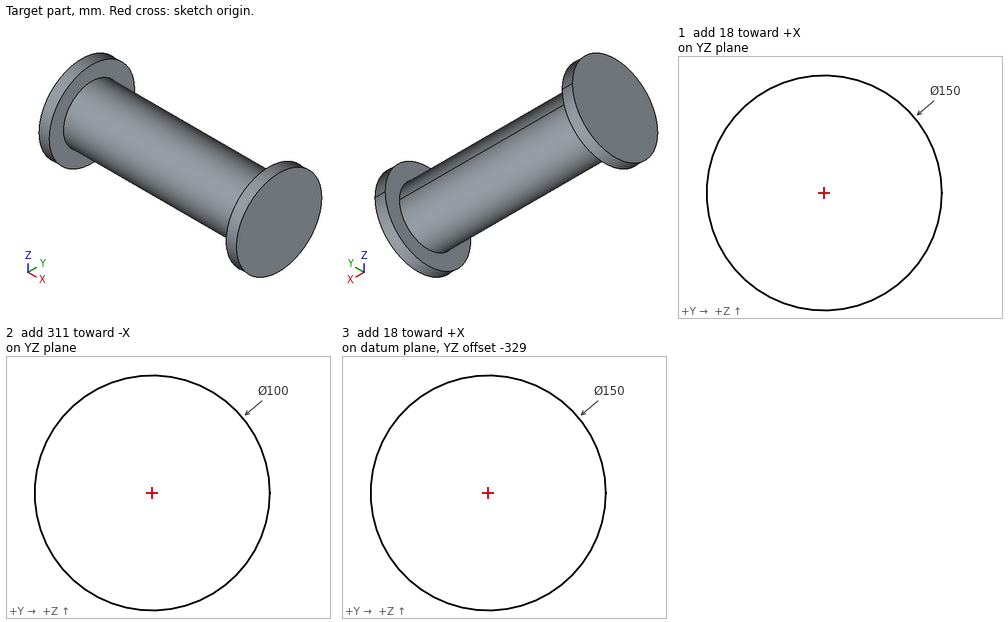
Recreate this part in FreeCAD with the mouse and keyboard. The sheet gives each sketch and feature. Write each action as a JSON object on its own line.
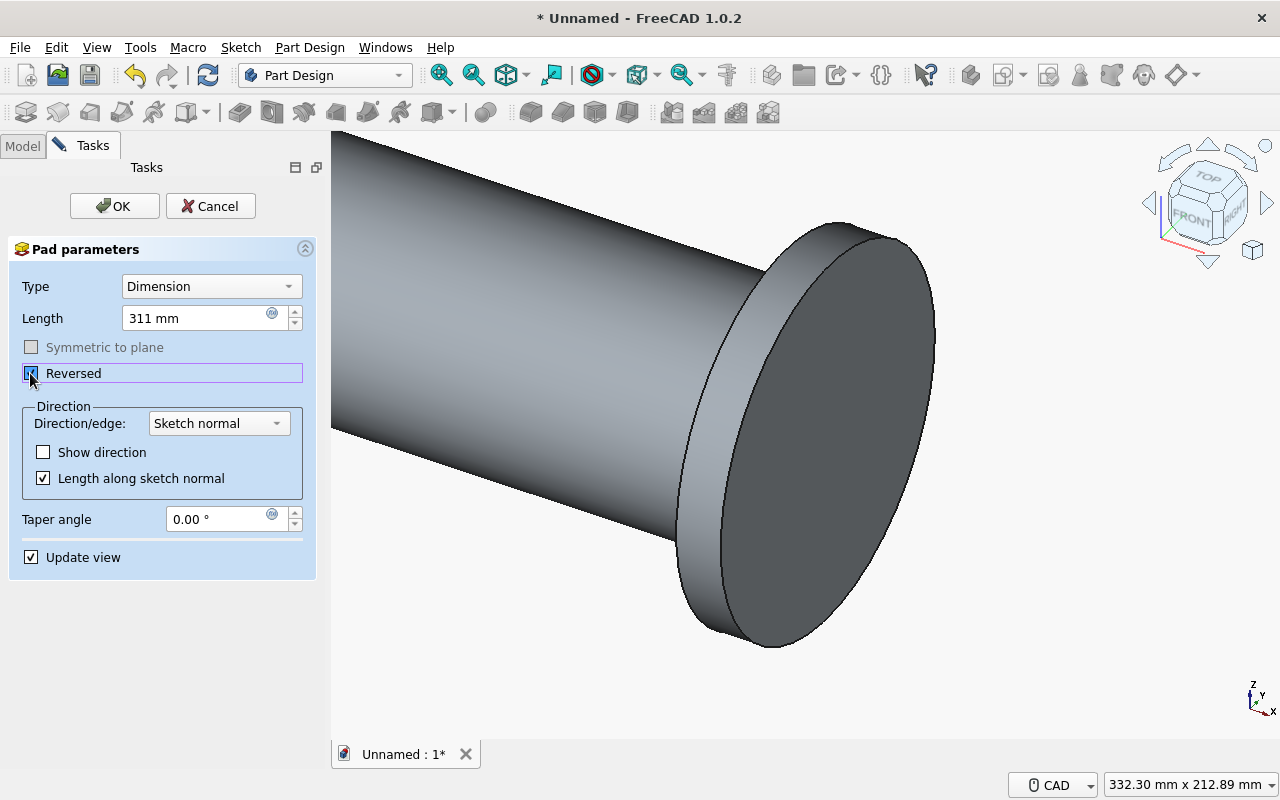
{"action": "left_click", "coordinate": [115, 206]}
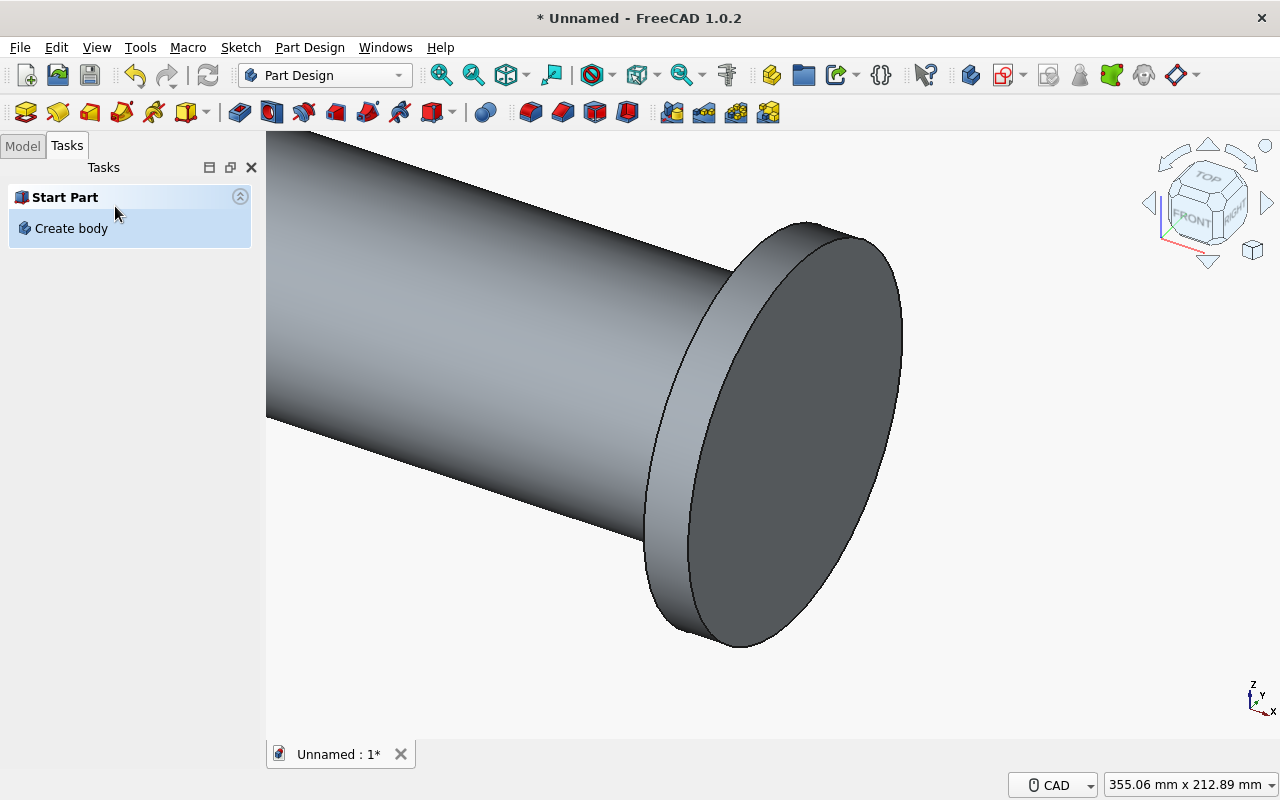
{"action": "left_click", "coordinate": [442, 76]}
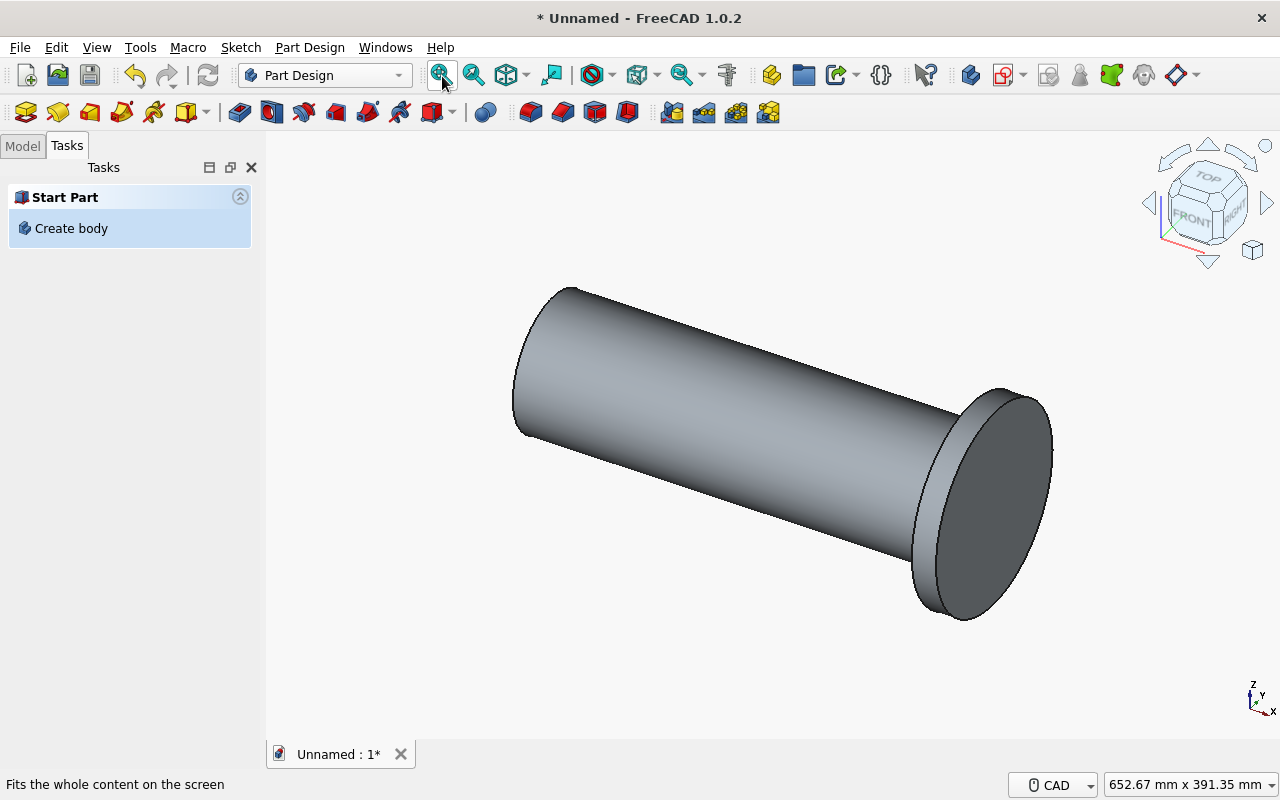
{"action": "left_click", "coordinate": [23, 145]}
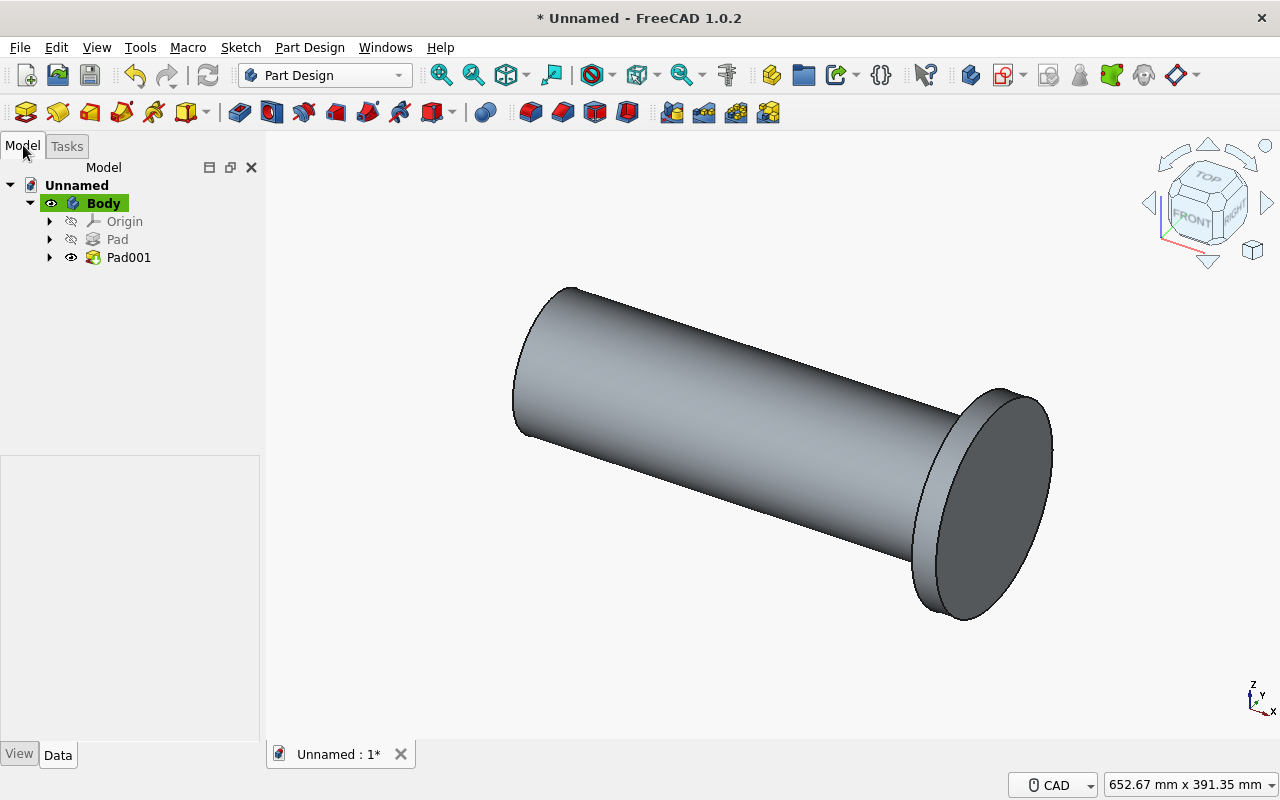
{"action": "left_click", "coordinate": [50, 221]}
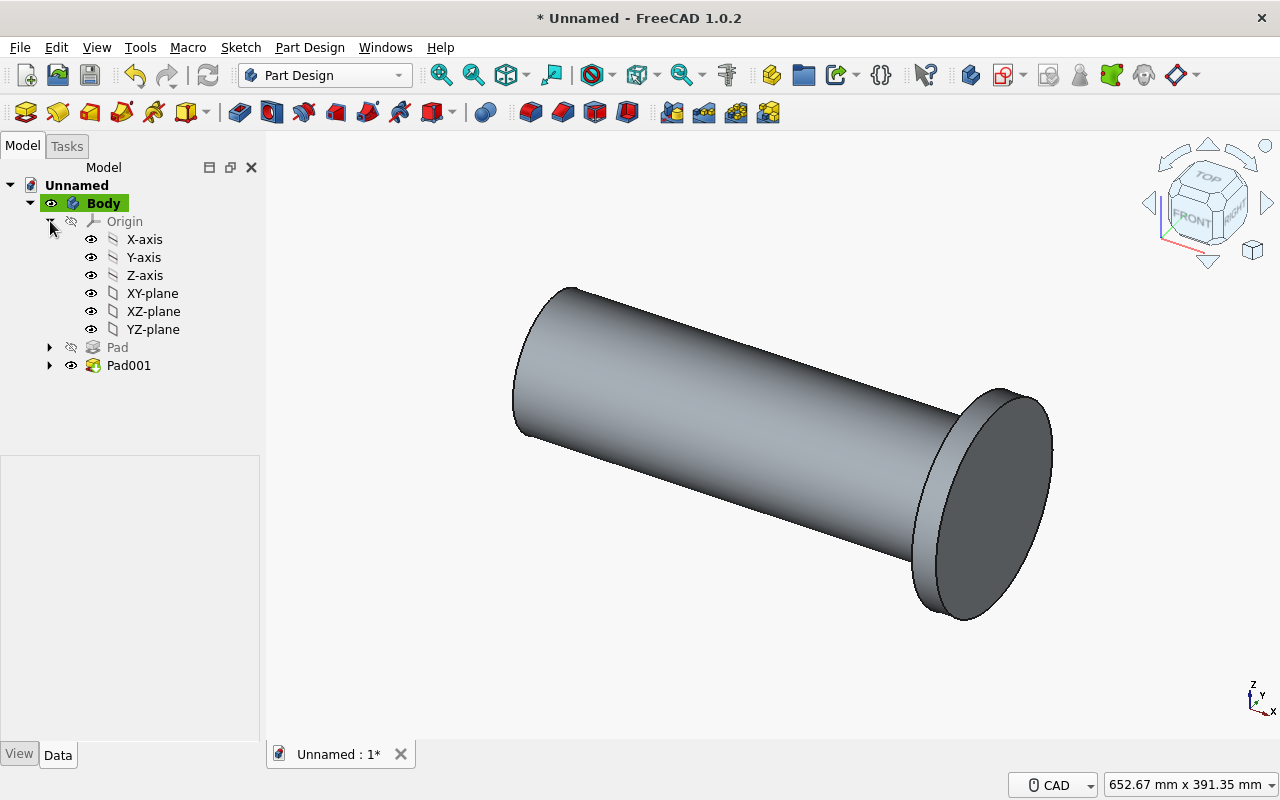
{"action": "left_click", "coordinate": [136, 329]}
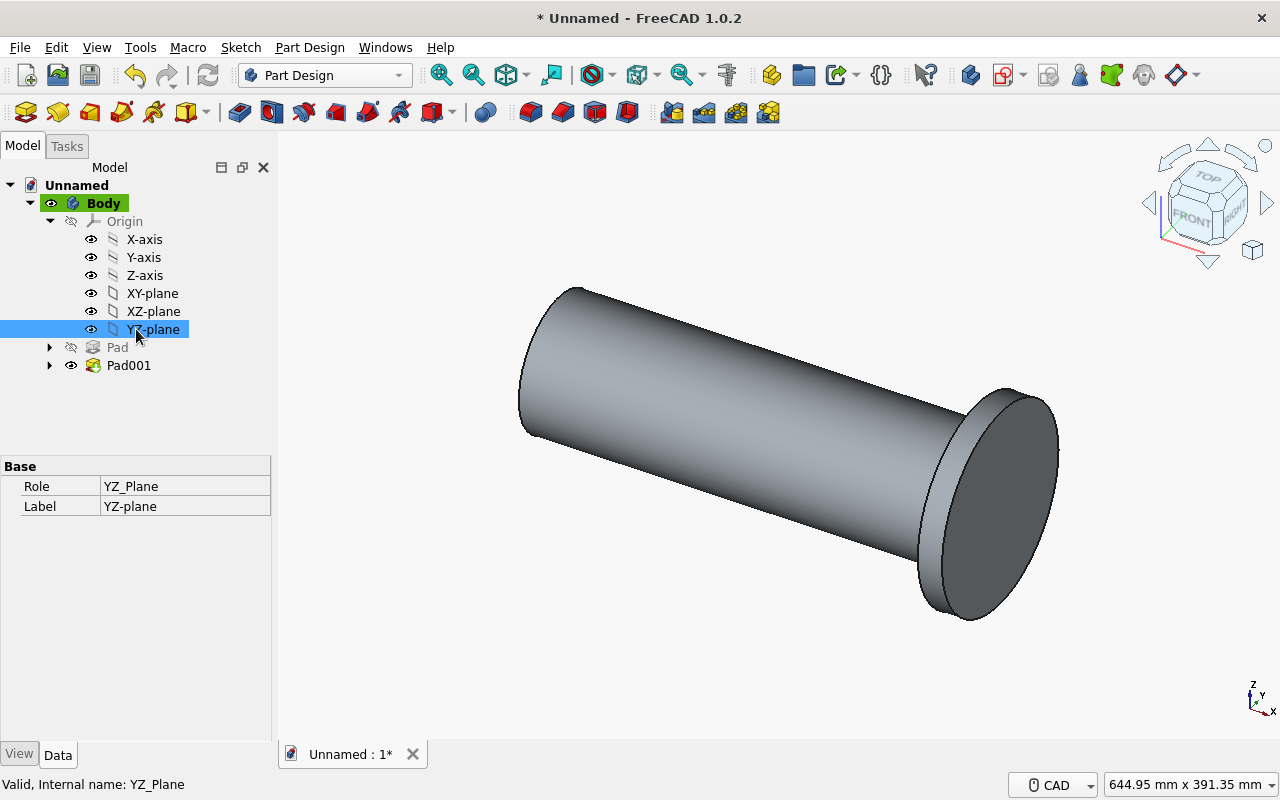
{"action": "left_click", "coordinate": [1176, 76]}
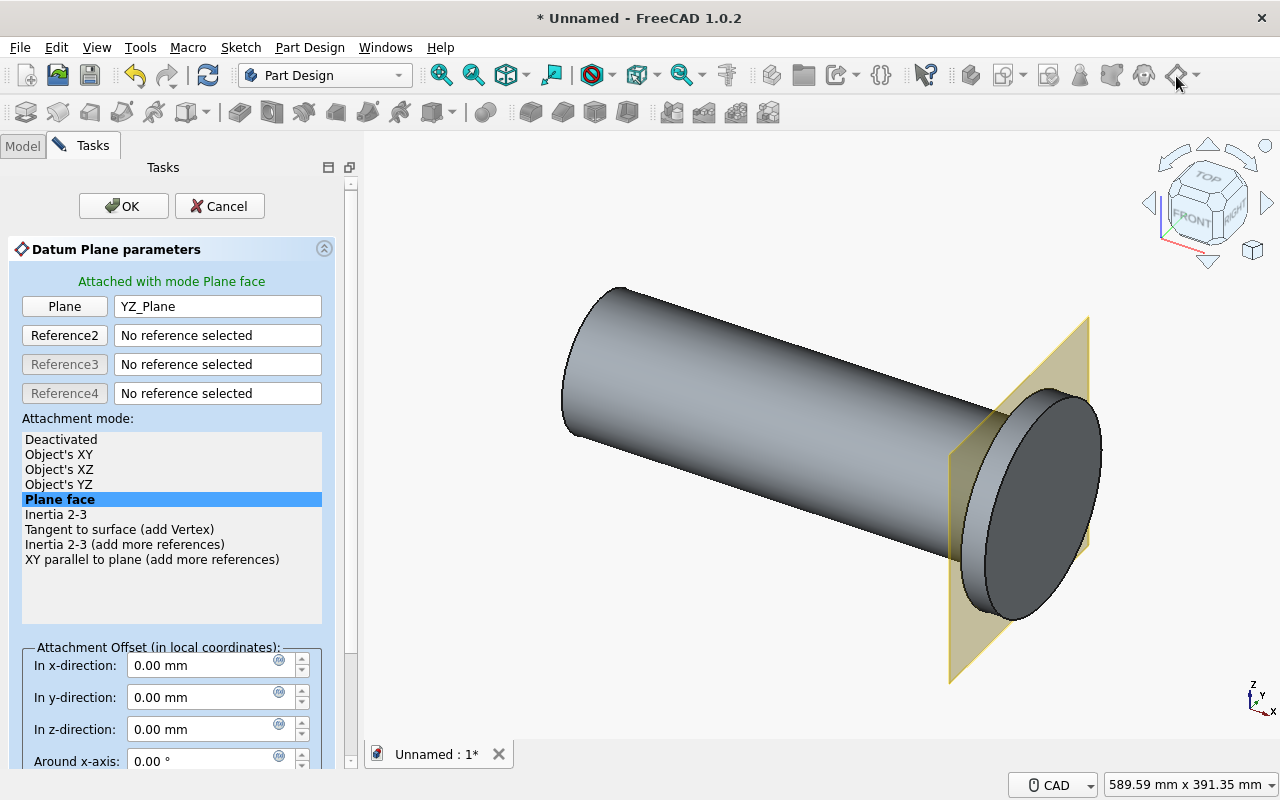
{"action": "triple_click", "coordinate": [210, 729]}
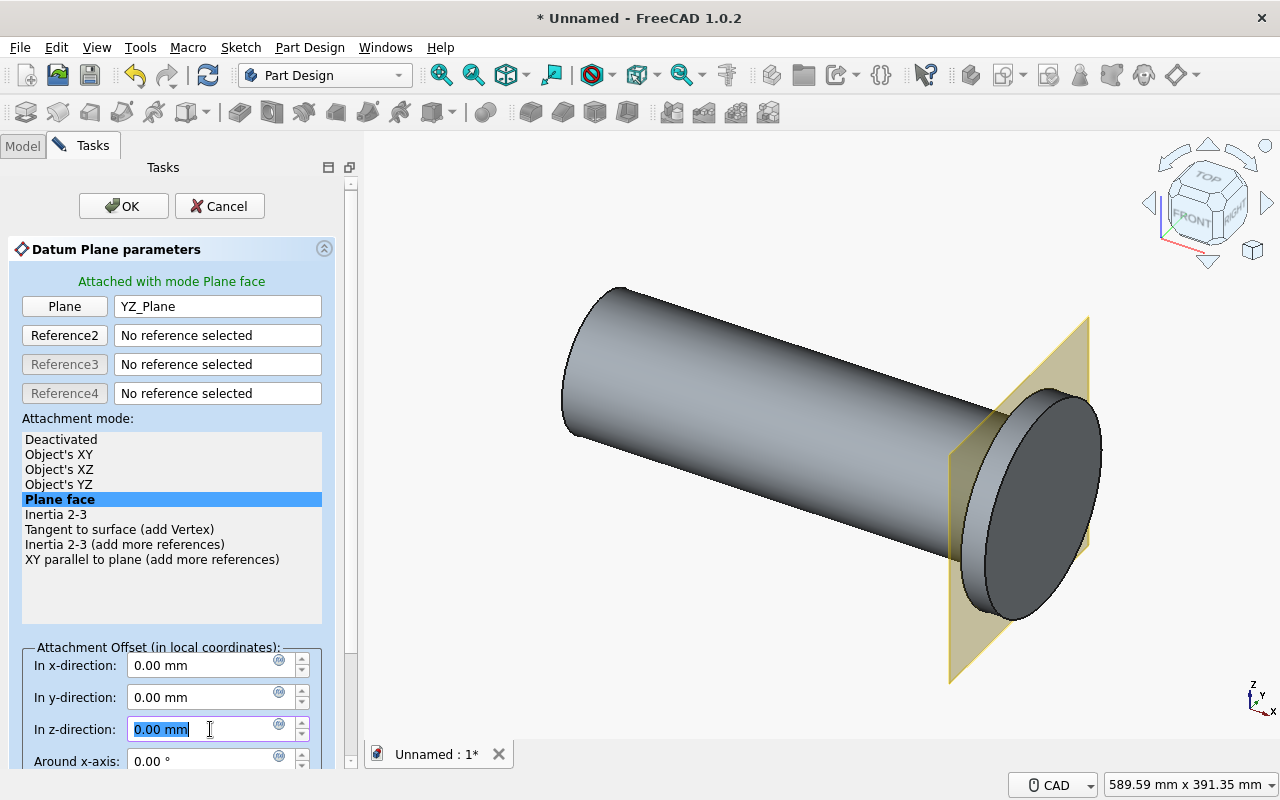
{"action": "type", "text": "-329"}
{"action": "key", "text": "Tab"}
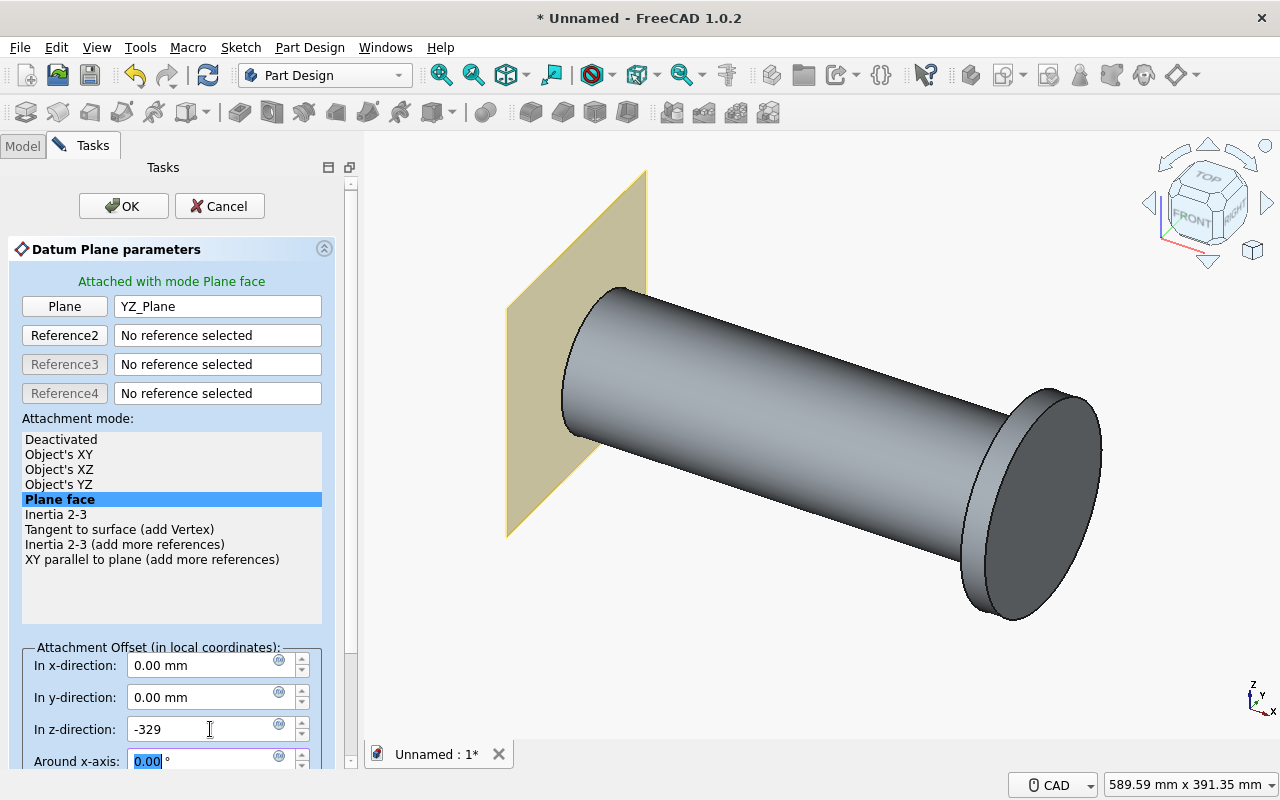
{"action": "left_click", "coordinate": [124, 206]}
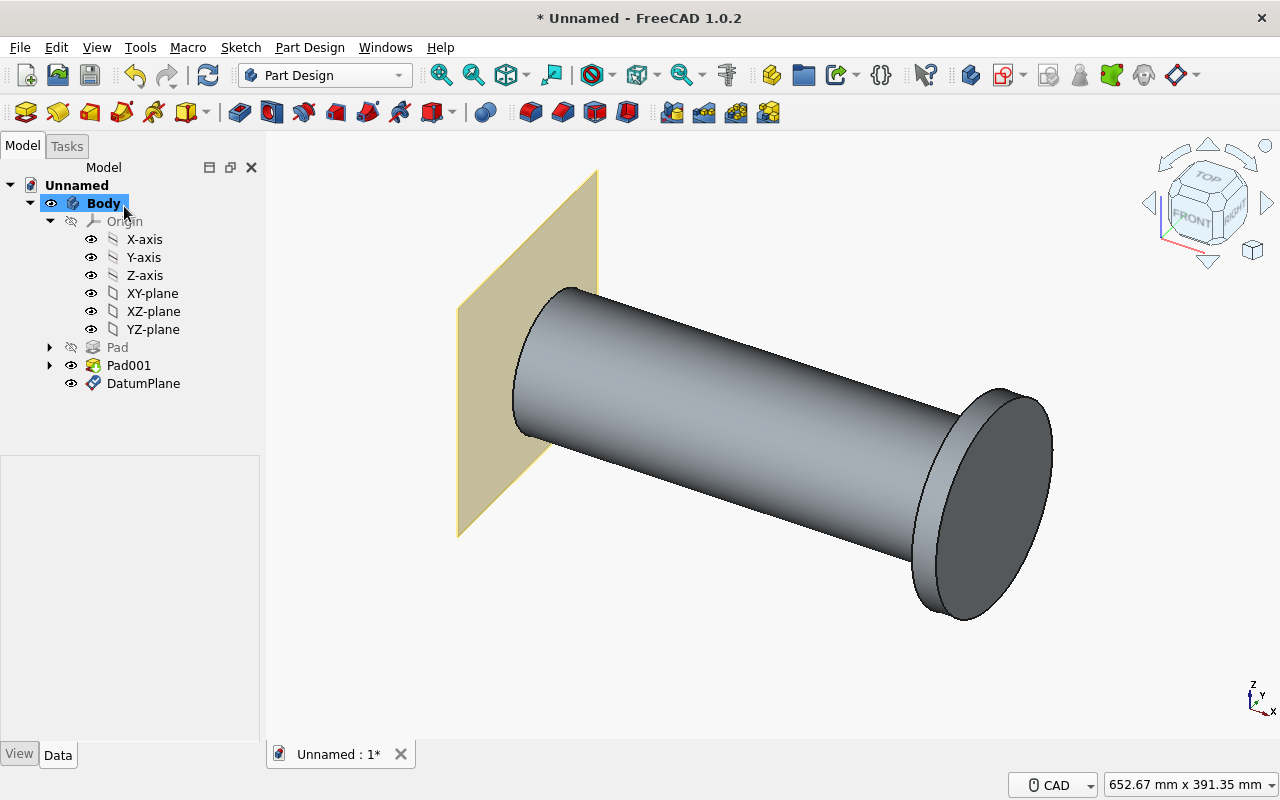
{"action": "left_click", "coordinate": [116, 383]}